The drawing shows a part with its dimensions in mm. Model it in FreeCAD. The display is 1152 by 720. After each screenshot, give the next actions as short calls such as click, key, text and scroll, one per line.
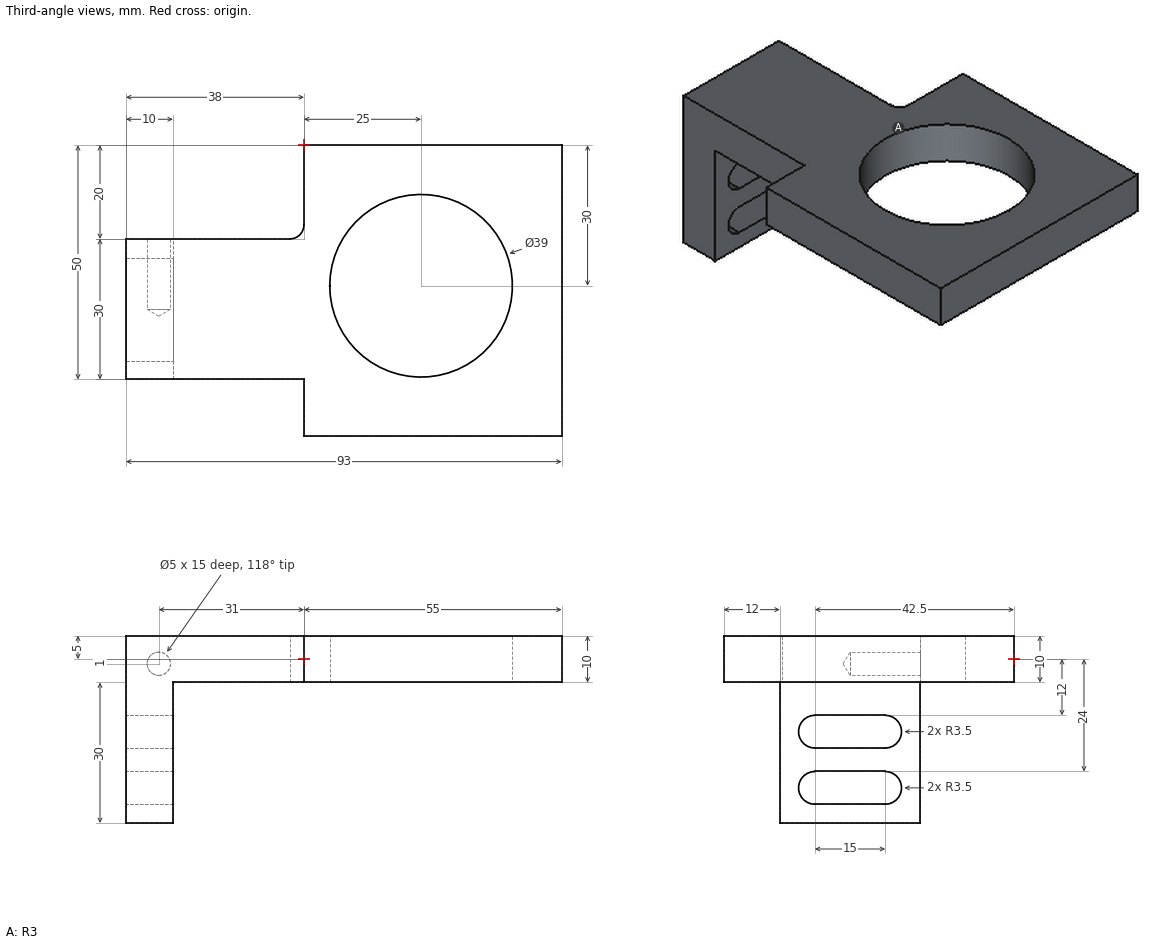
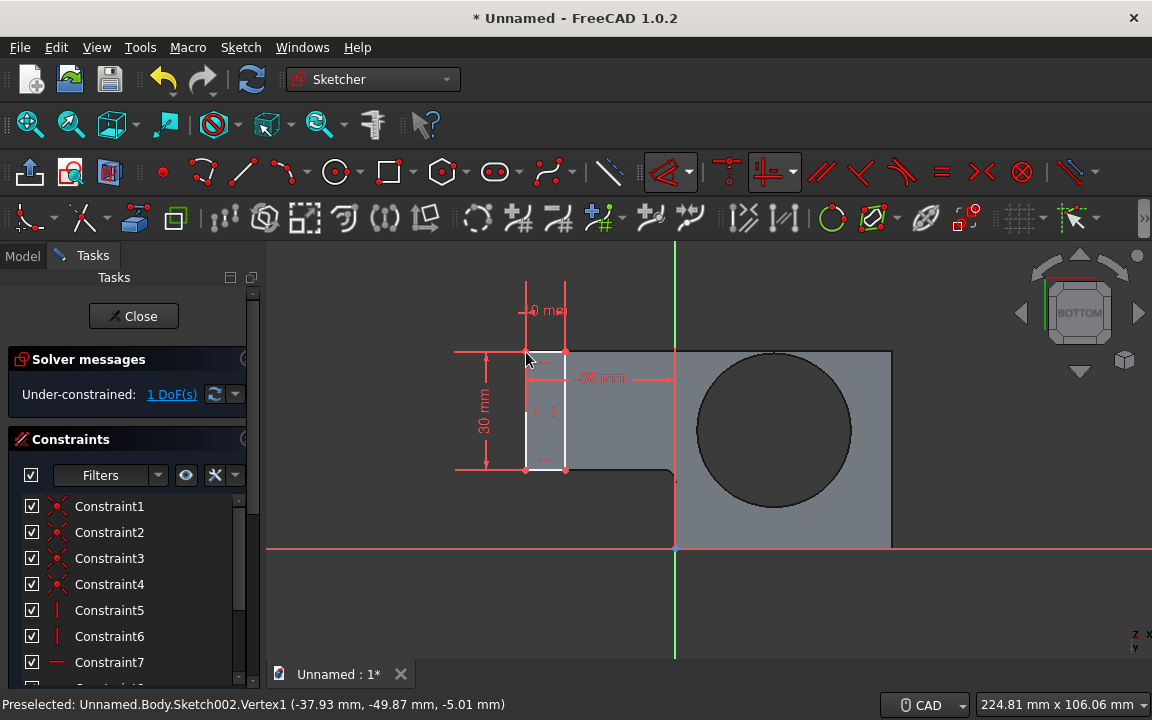
click(526, 352)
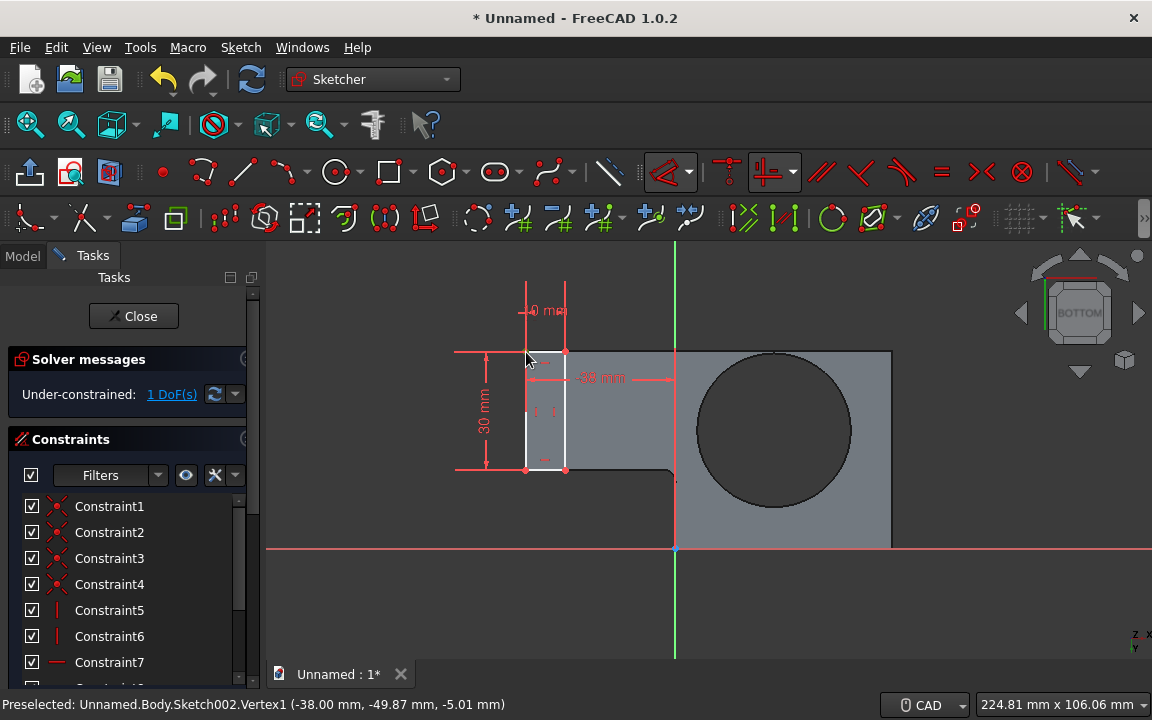
click(692, 172)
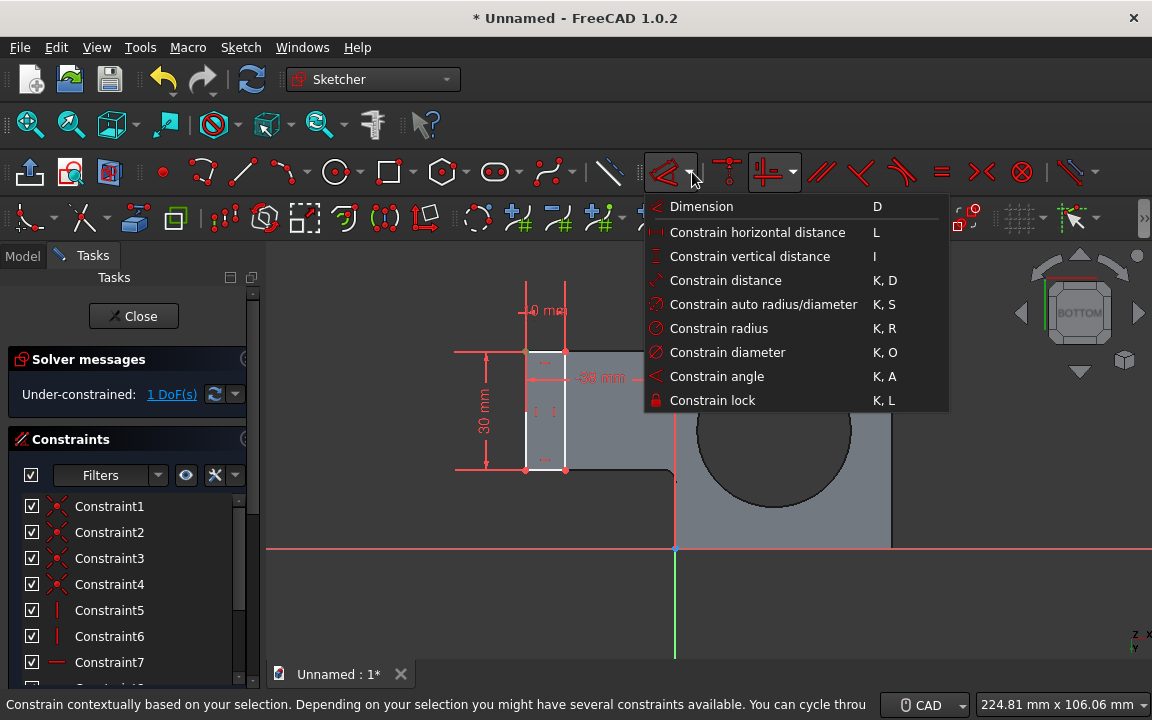
click(797, 256)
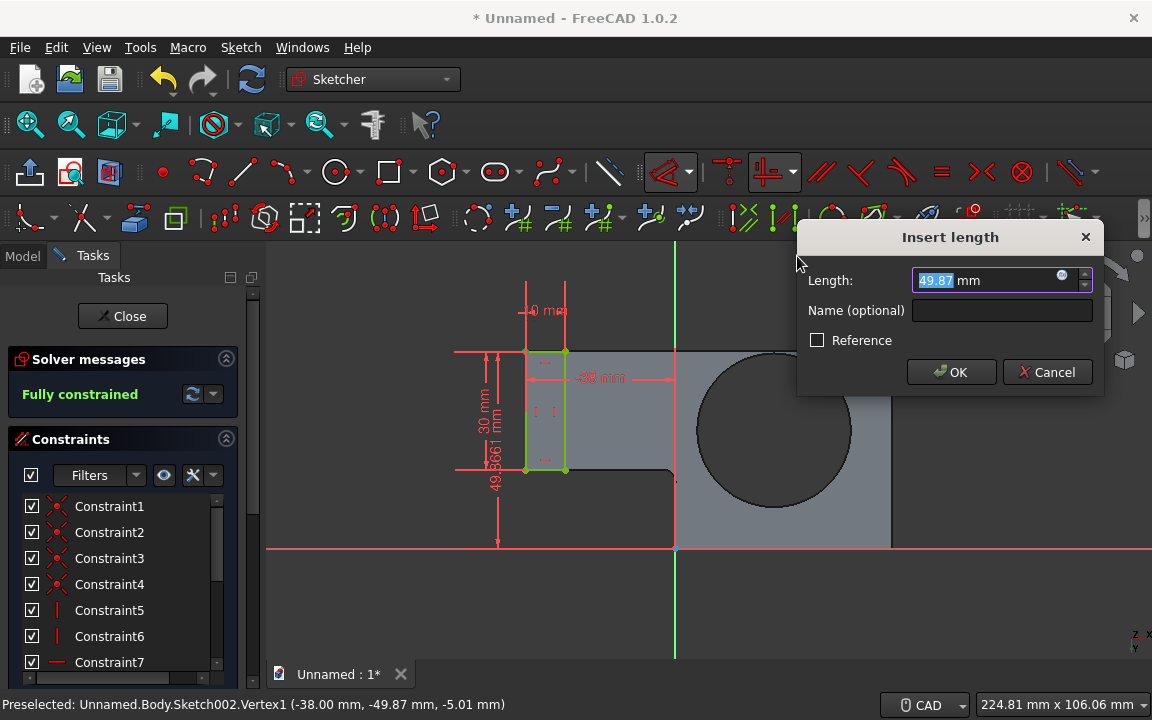
text(50)
key(Return)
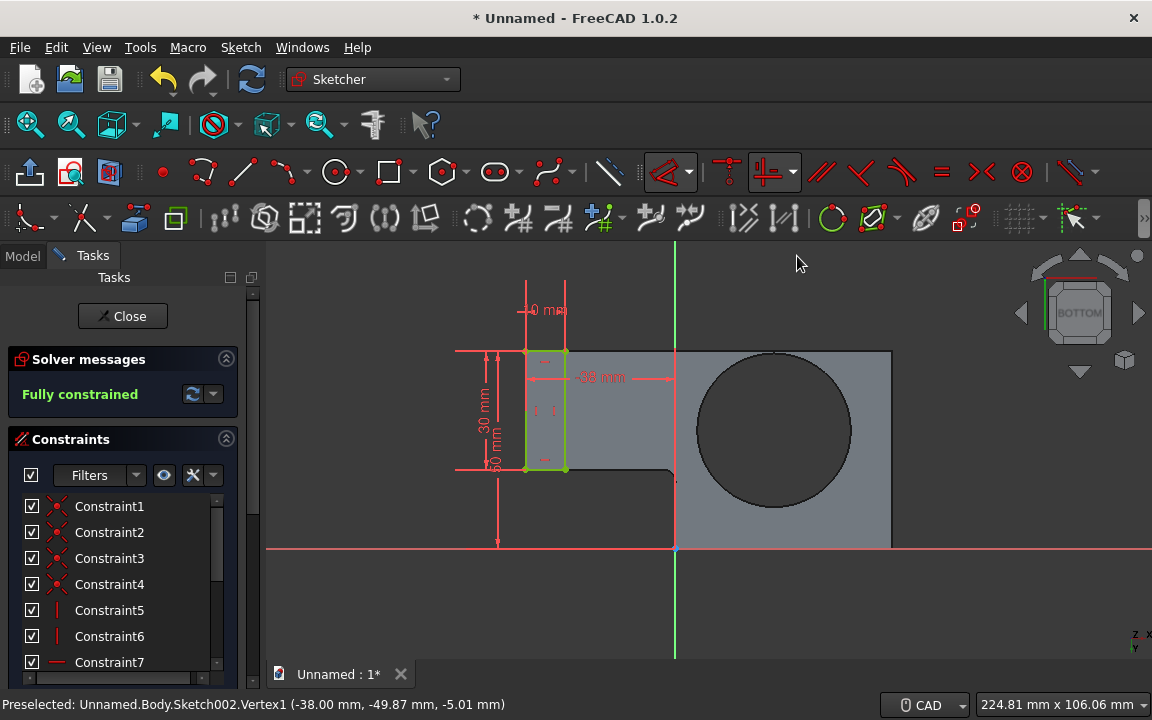
click(123, 316)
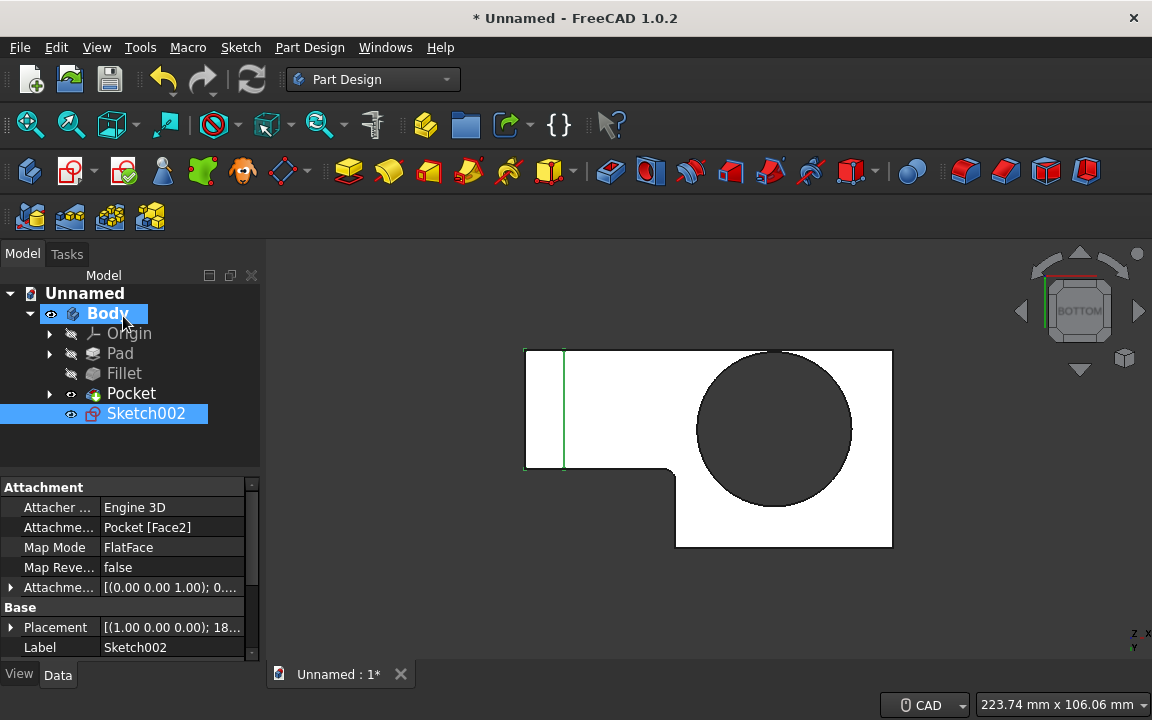
click(350, 172)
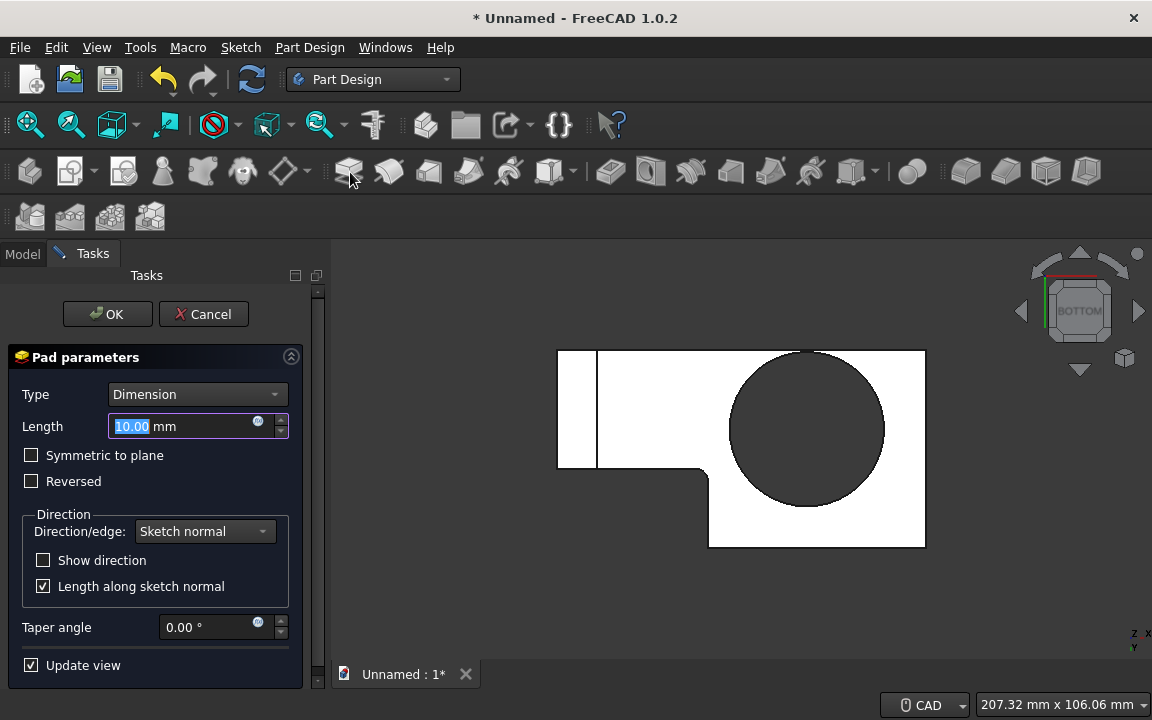
text(30)
key(Tab)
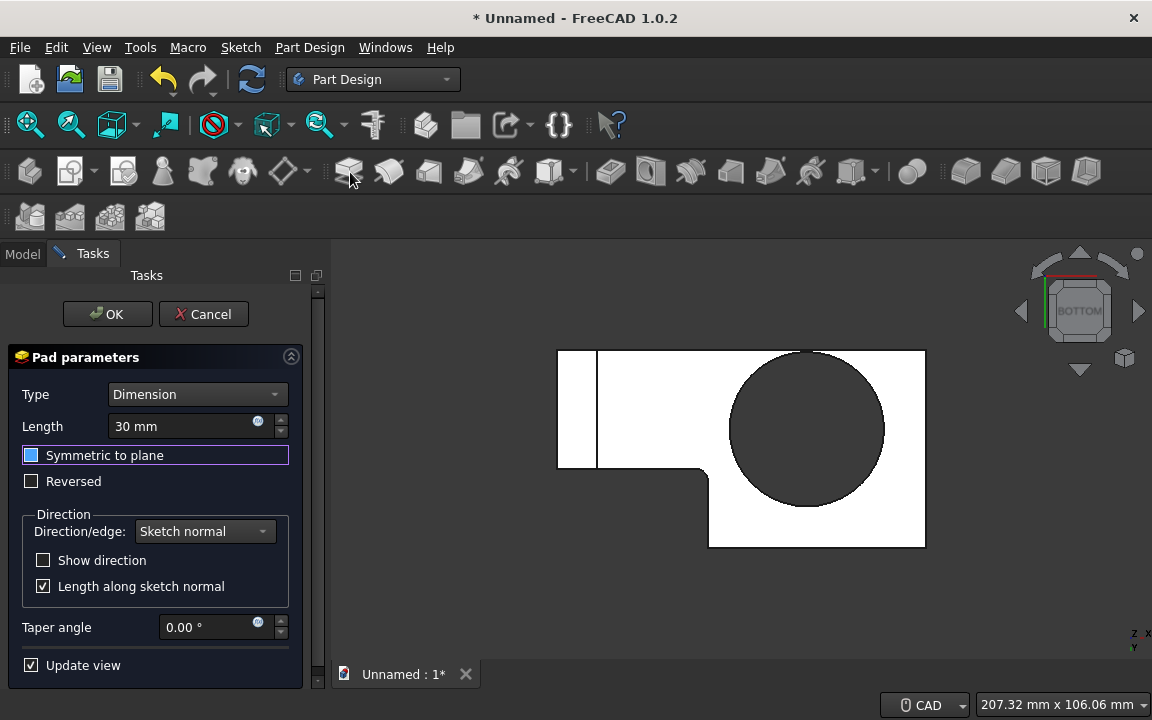
click(108, 314)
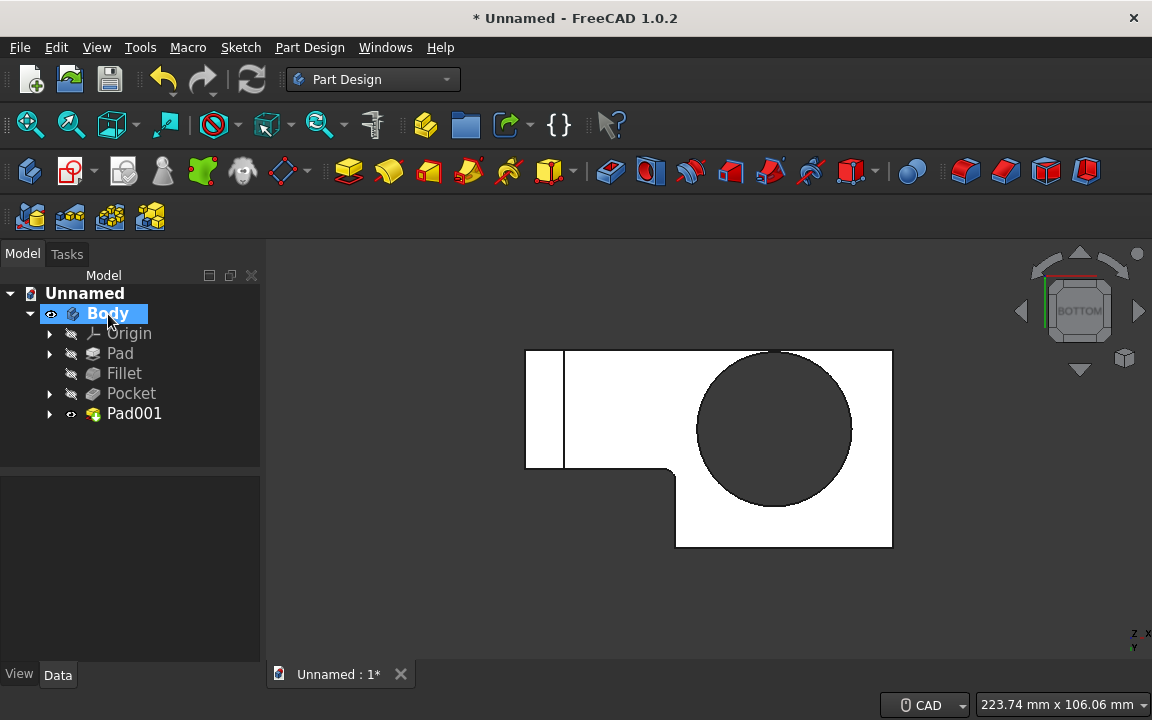
key(0)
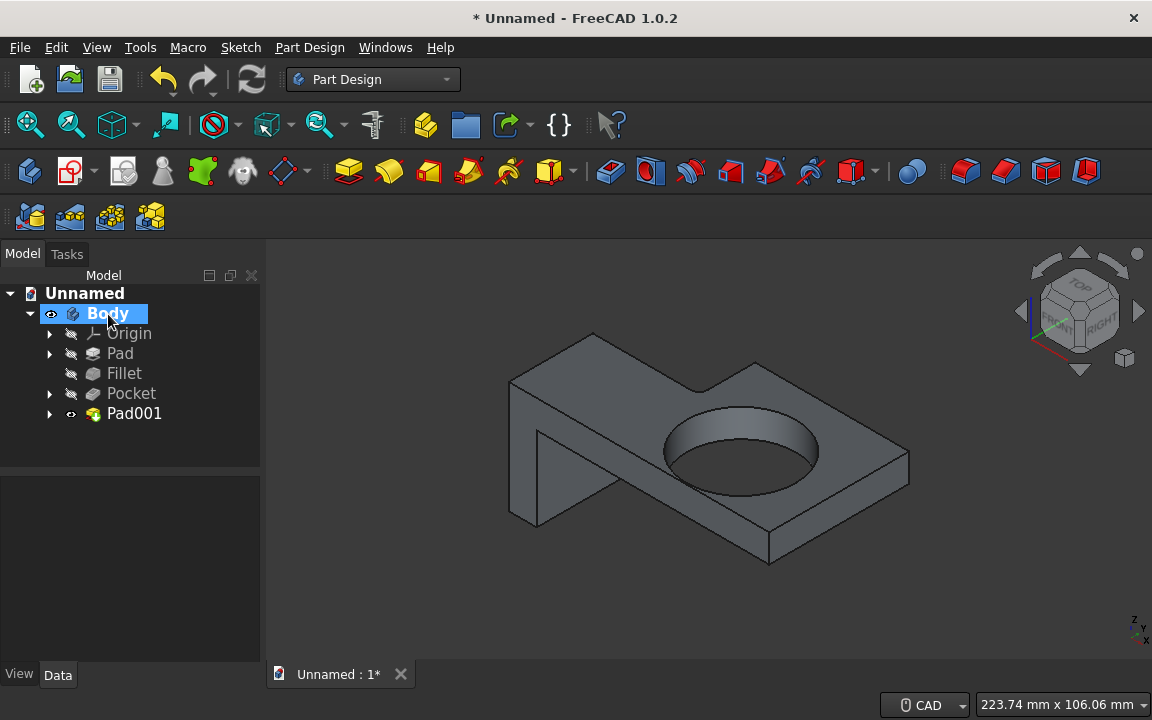
key(v)
key(f)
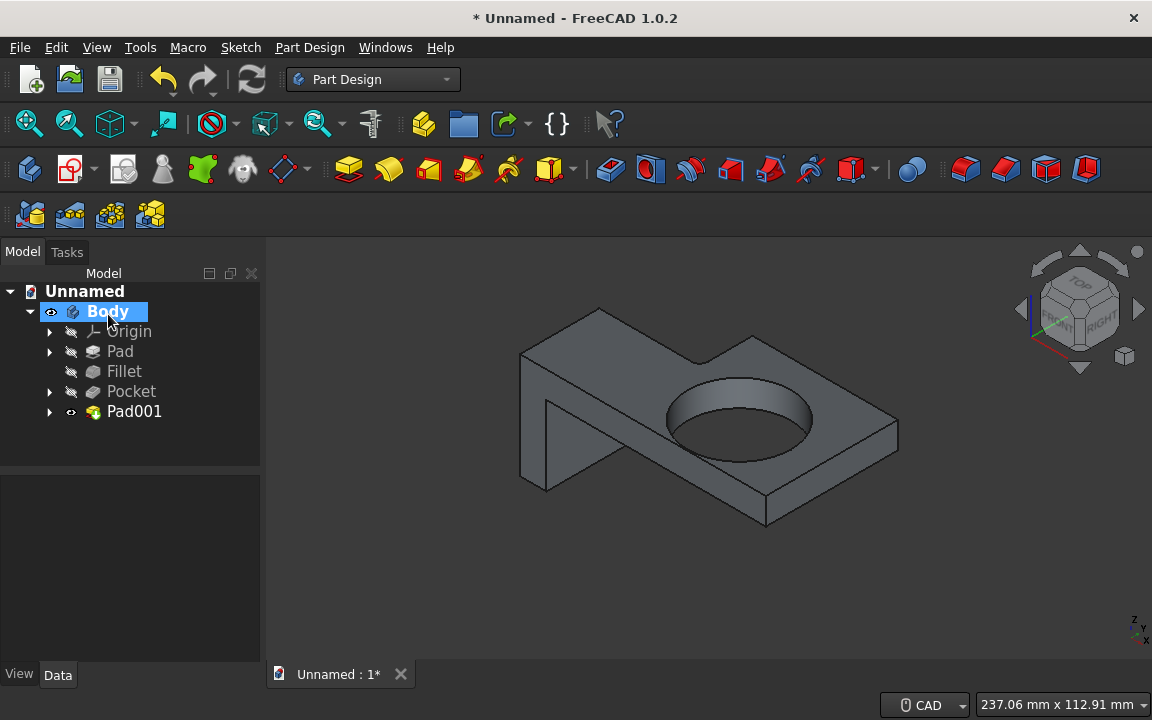
click(586, 435)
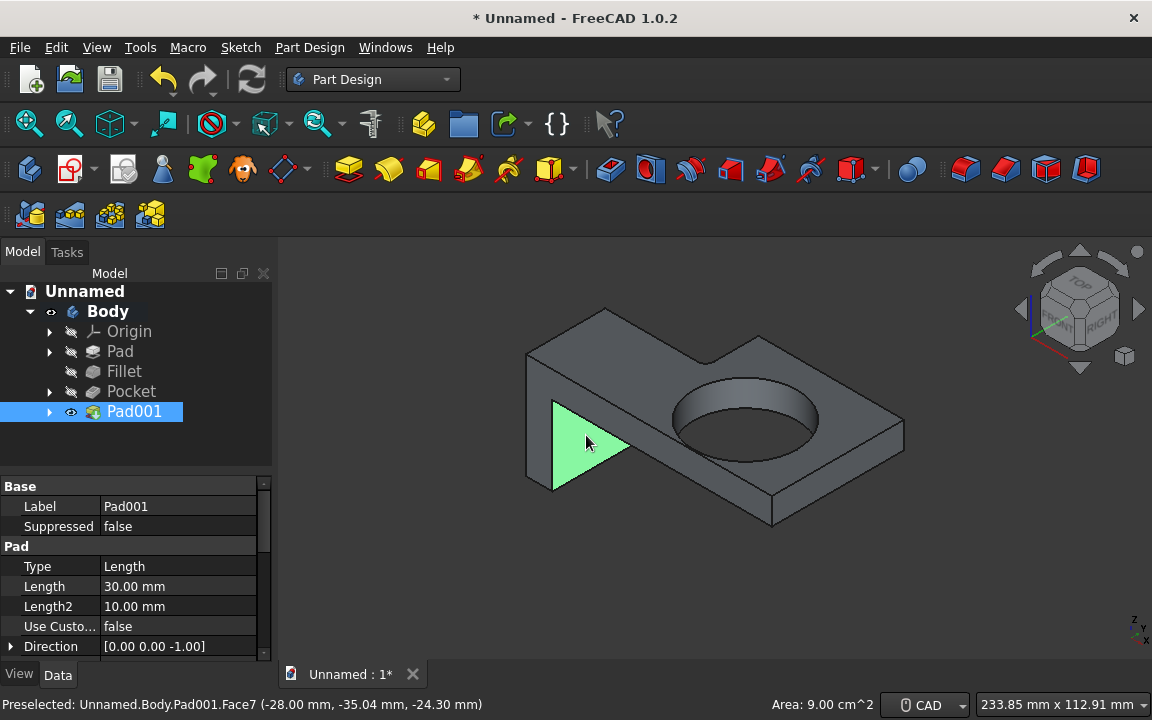
click(70, 170)